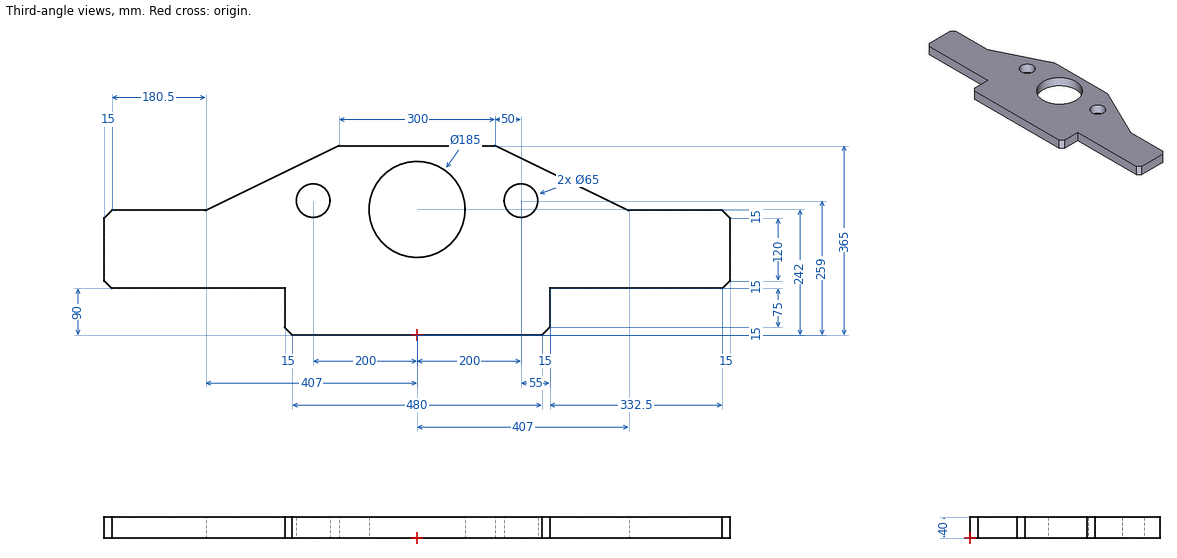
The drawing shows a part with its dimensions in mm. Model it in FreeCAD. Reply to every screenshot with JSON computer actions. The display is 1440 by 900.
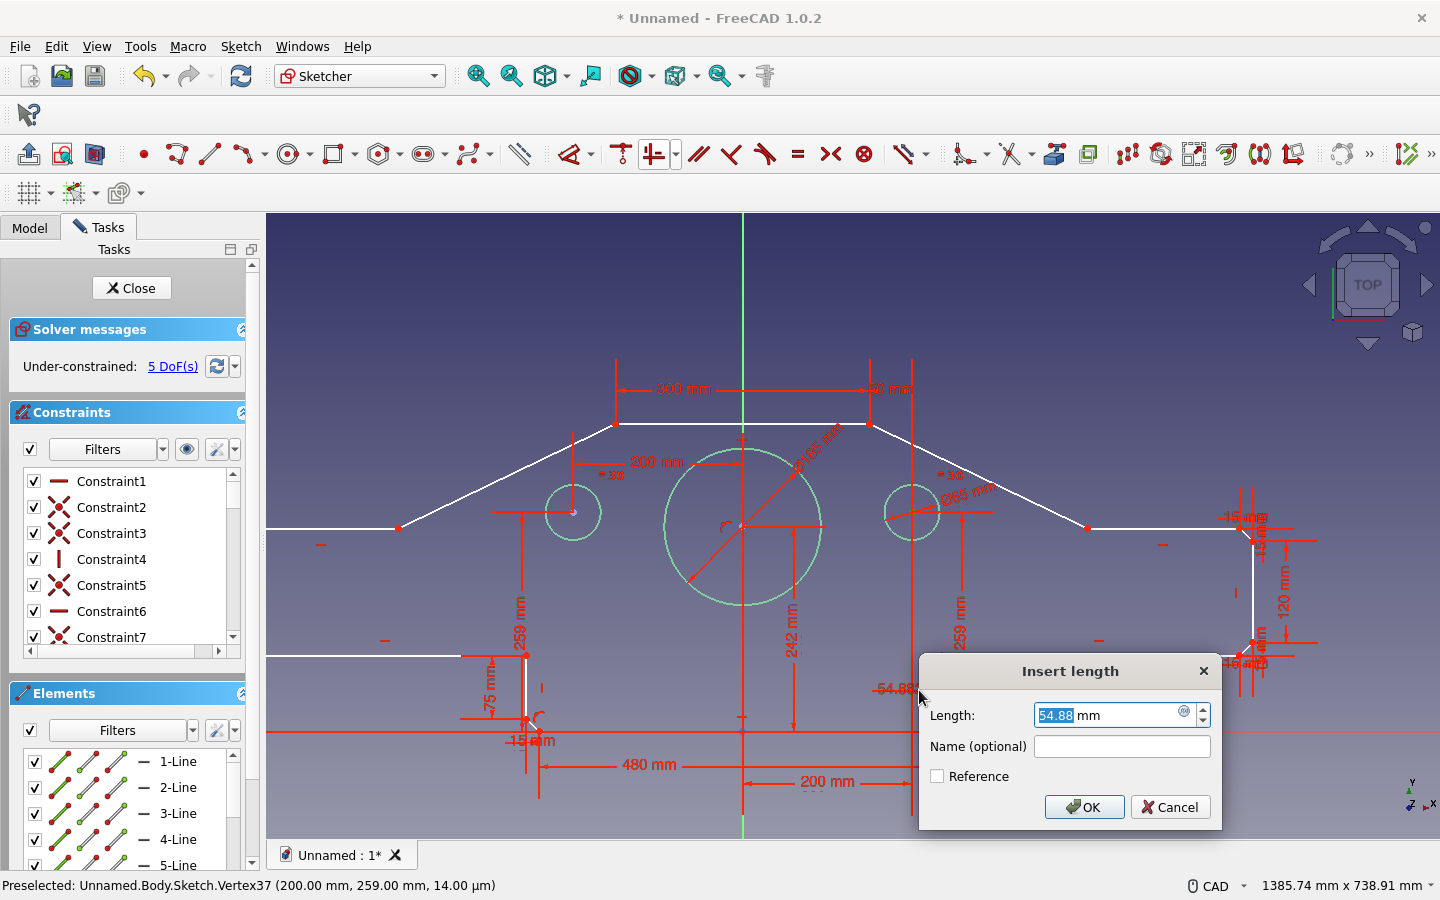
{"action": "type", "text": "55"}
{"action": "key", "text": "Return"}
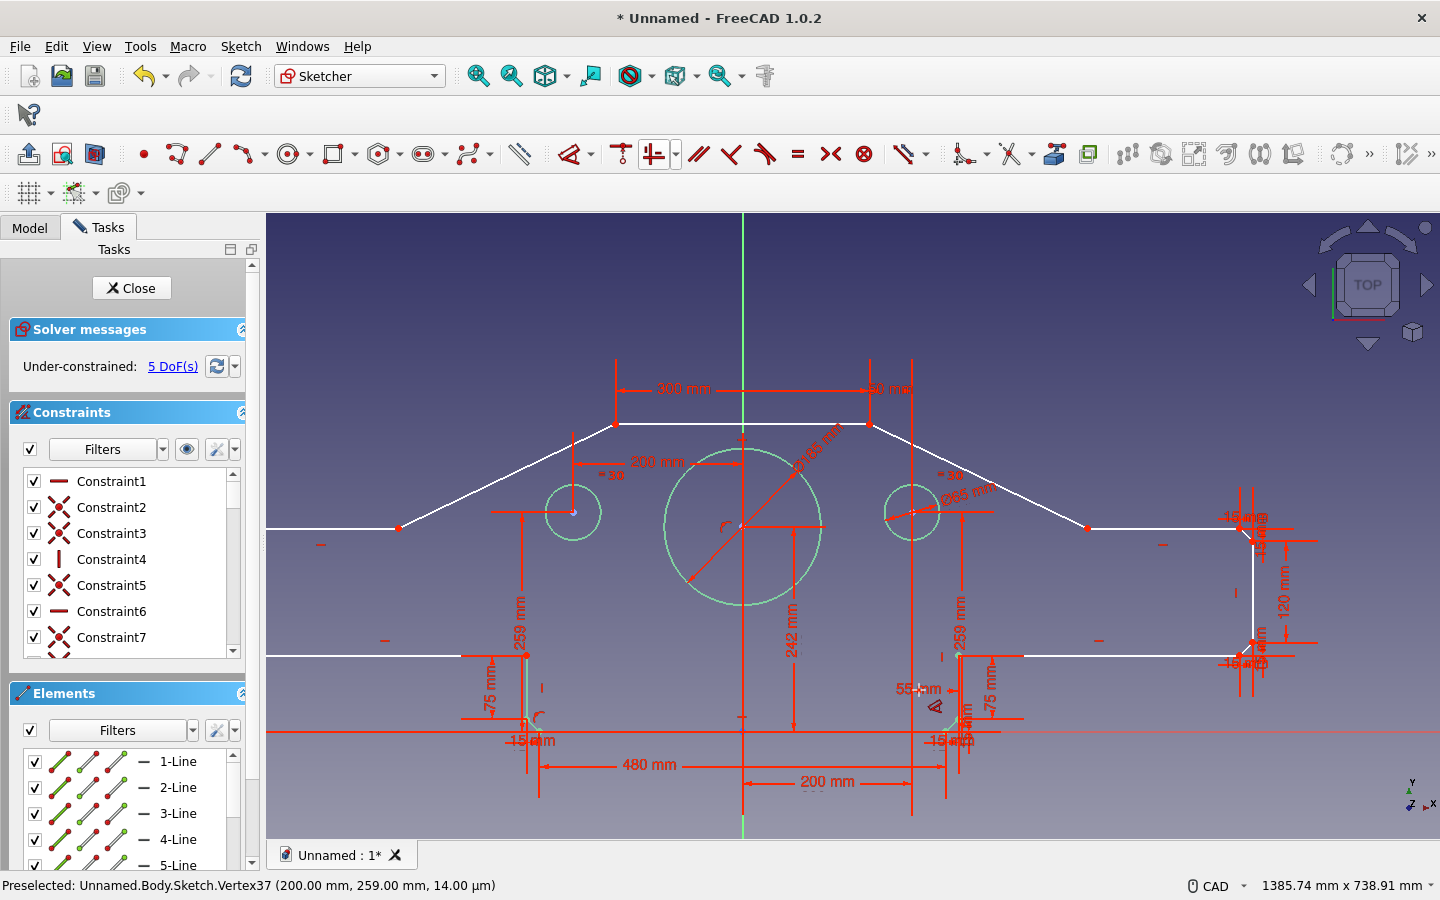
{"action": "left_click", "coordinate": [1088, 529]}
{"action": "left_click", "coordinate": [915, 766]}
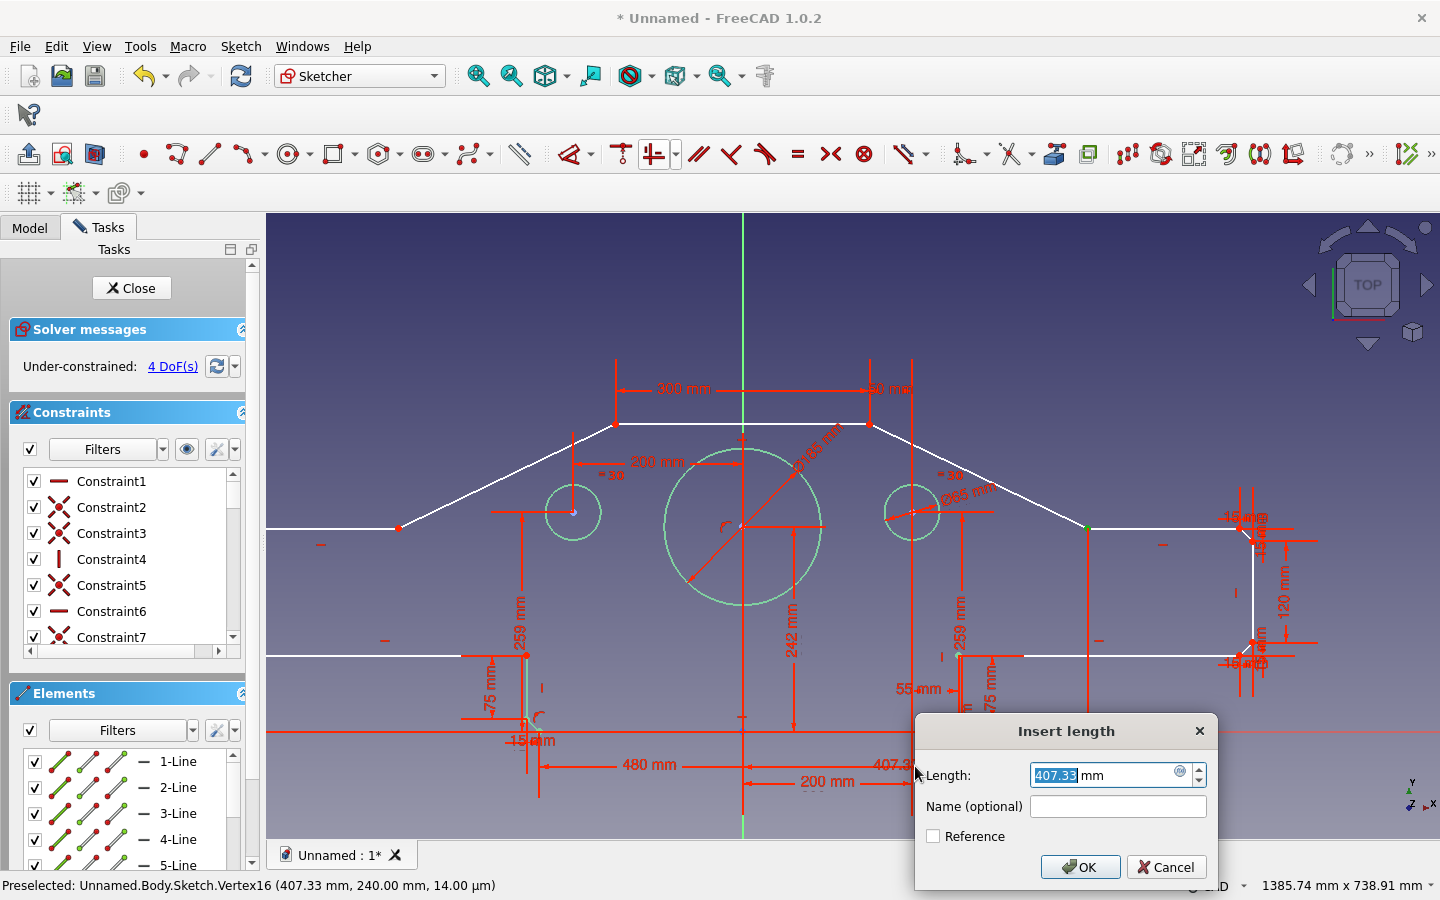
{"action": "type", "text": "407"}
{"action": "key", "text": "Return"}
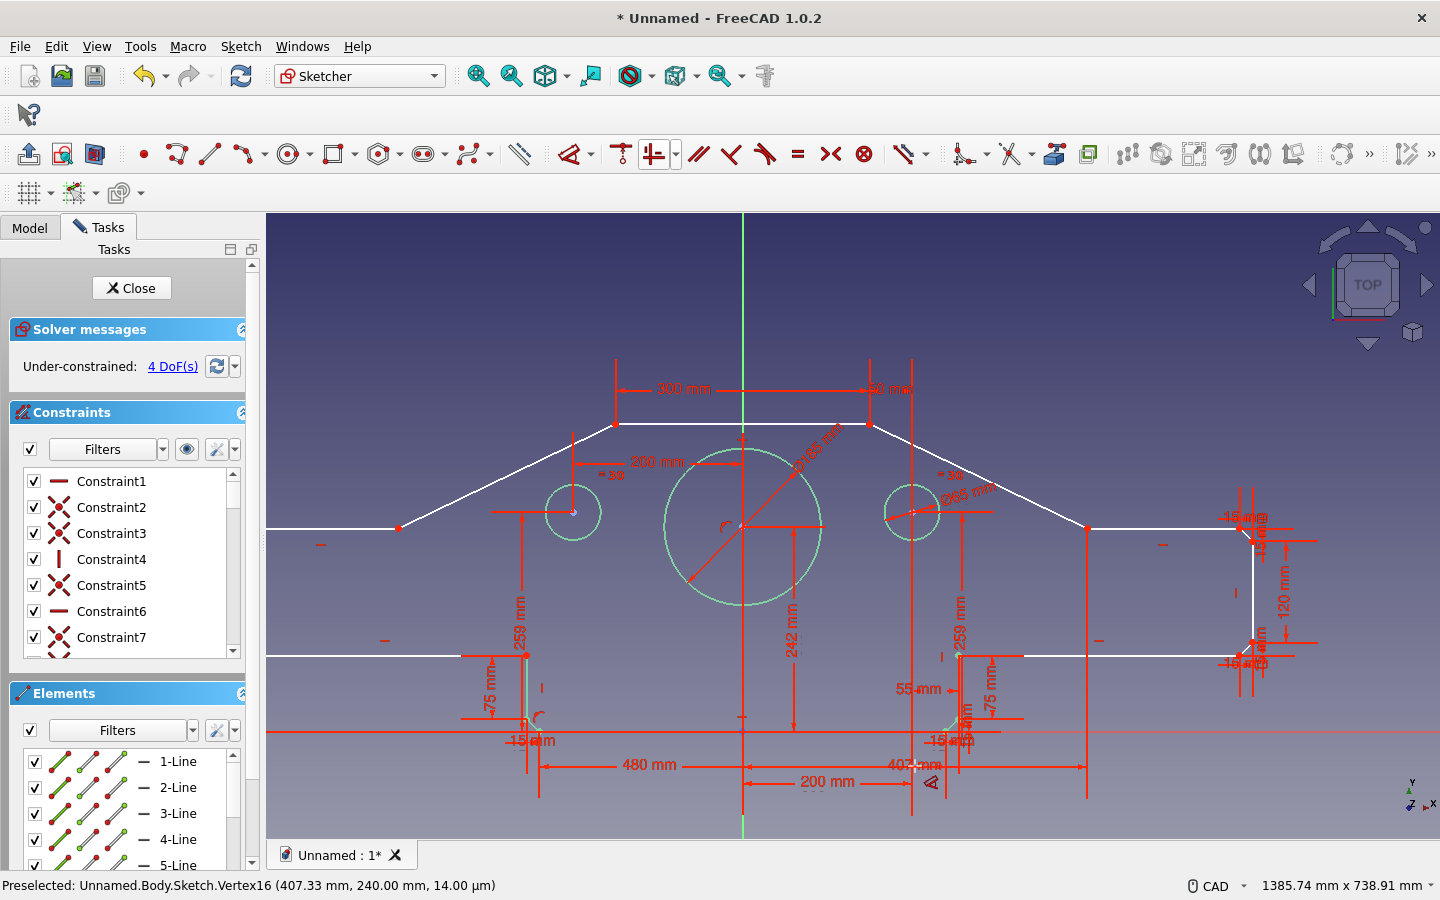
{"action": "left_click", "coordinate": [870, 424]}
{"action": "left_click", "coordinate": [904, 578]}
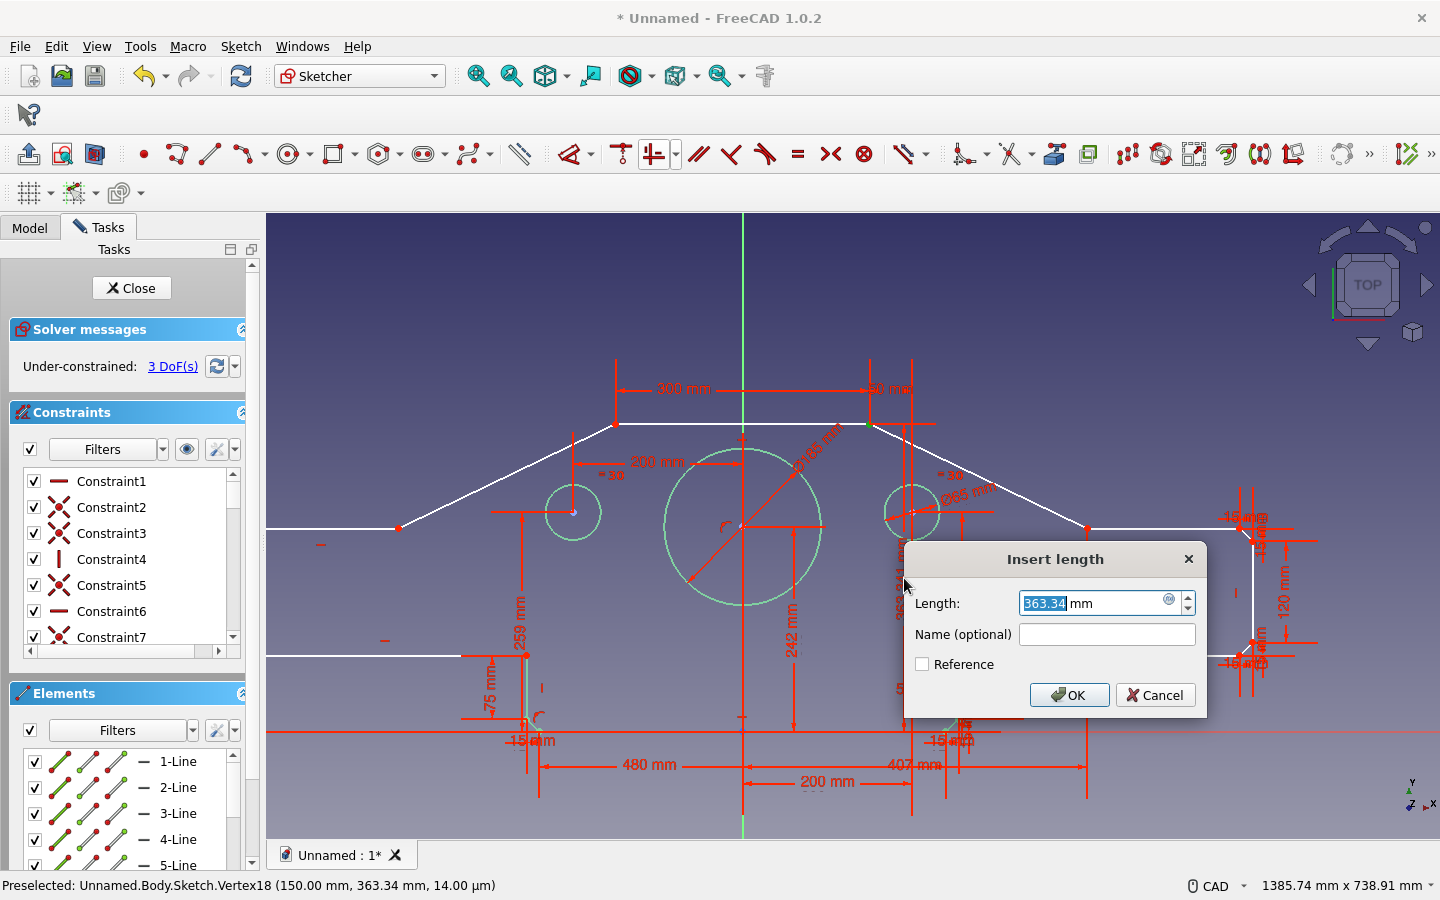
{"action": "type", "text": "365"}
{"action": "key", "text": "Return"}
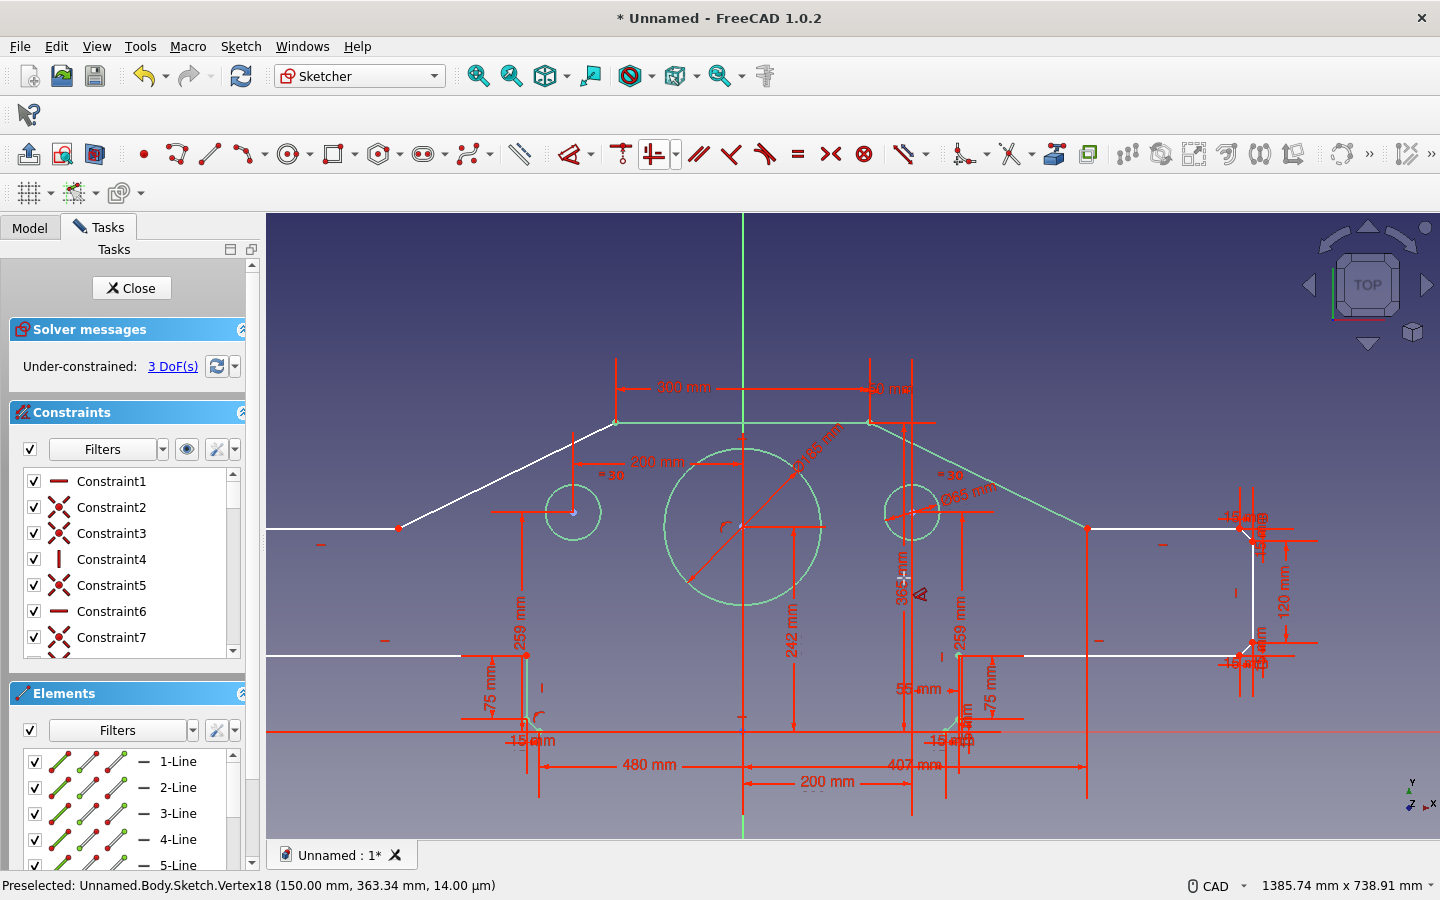
{"action": "left_click", "coordinate": [399, 529]}
{"action": "left_click", "coordinate": [571, 766]}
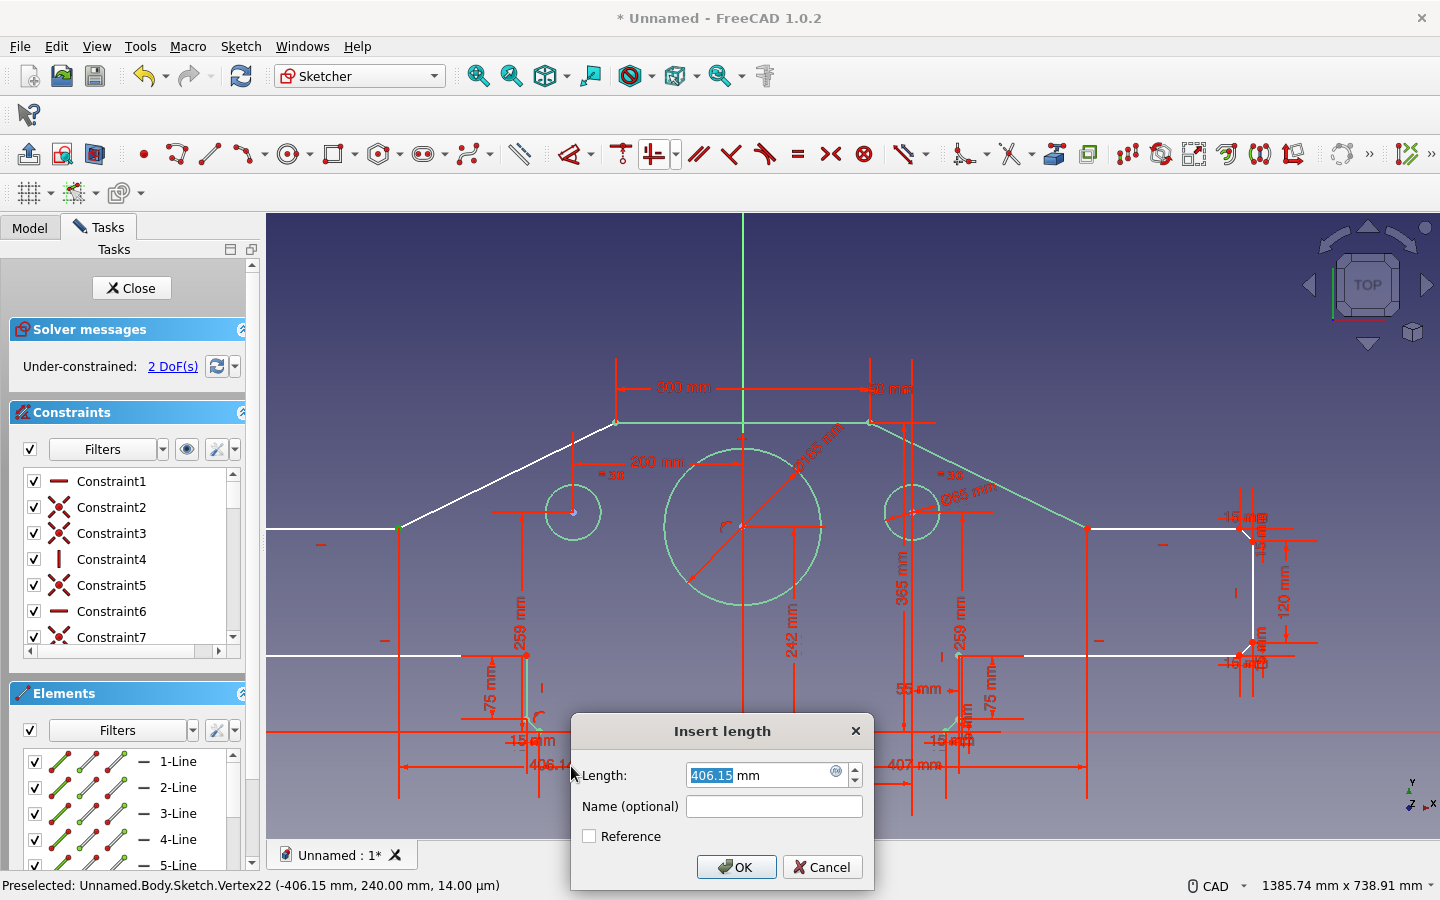
{"action": "type", "text": "407"}
{"action": "key", "text": "Return"}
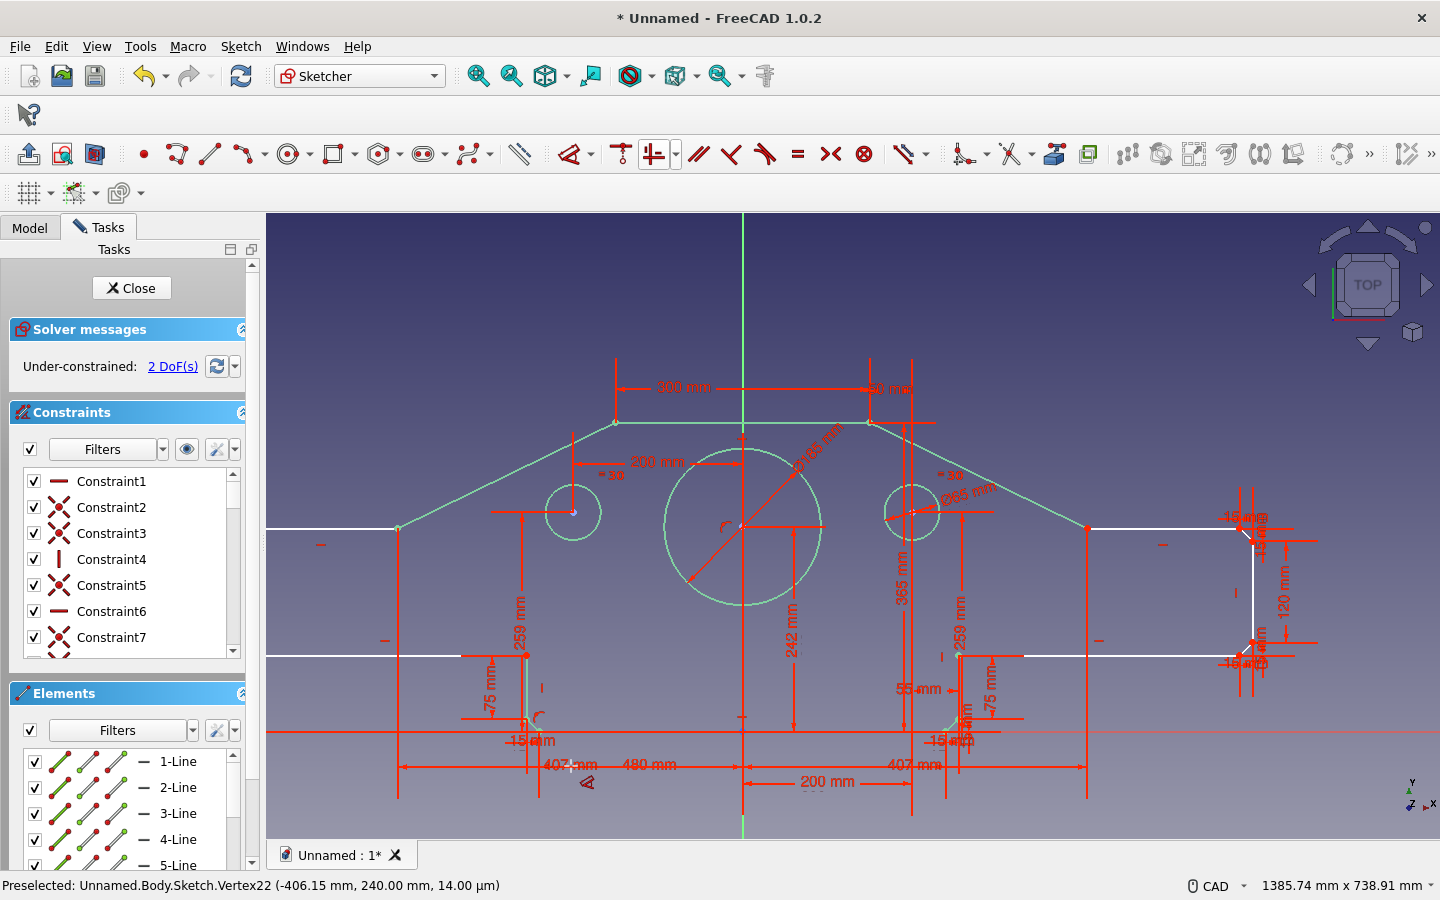
{"action": "left_click", "coordinate": [1043, 656]}
{"action": "left_click", "coordinate": [1099, 690]}